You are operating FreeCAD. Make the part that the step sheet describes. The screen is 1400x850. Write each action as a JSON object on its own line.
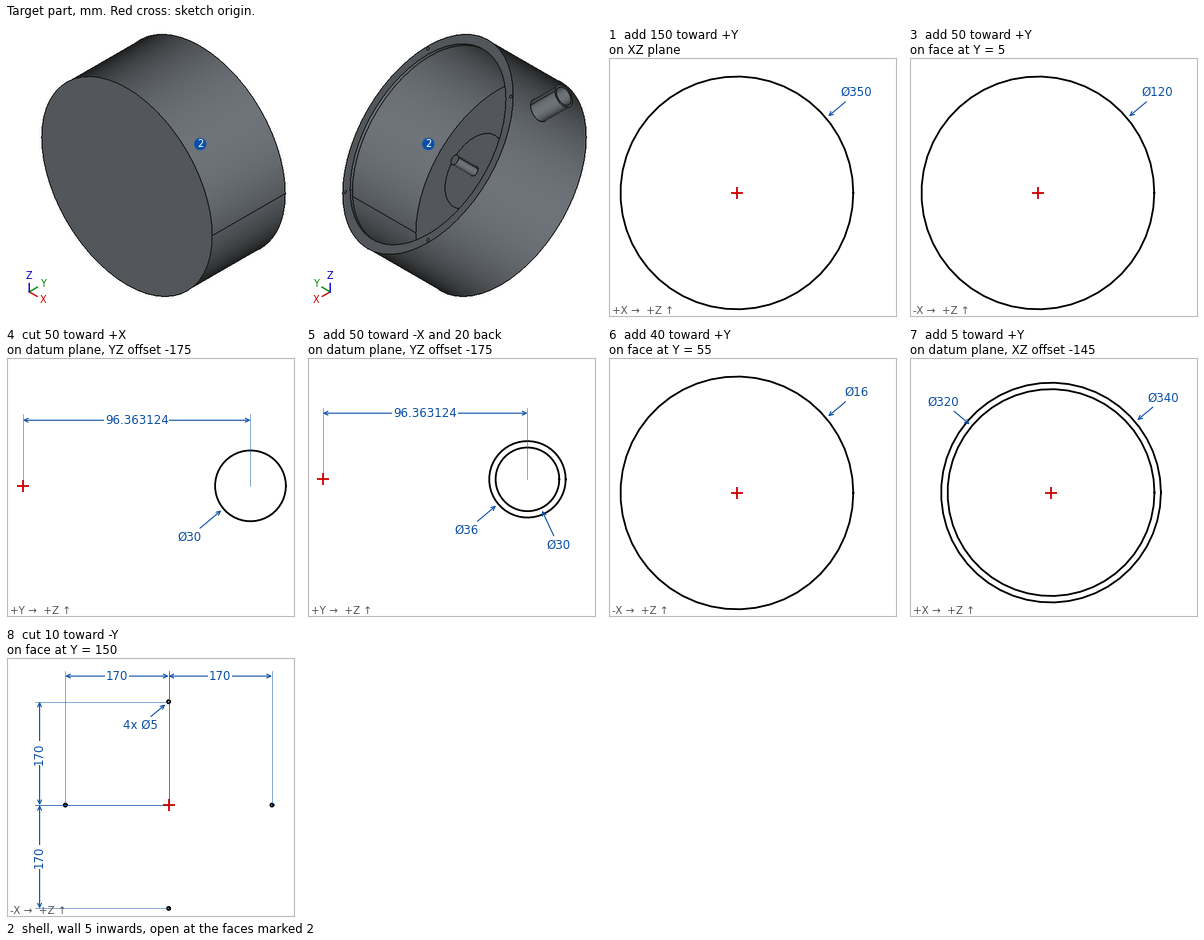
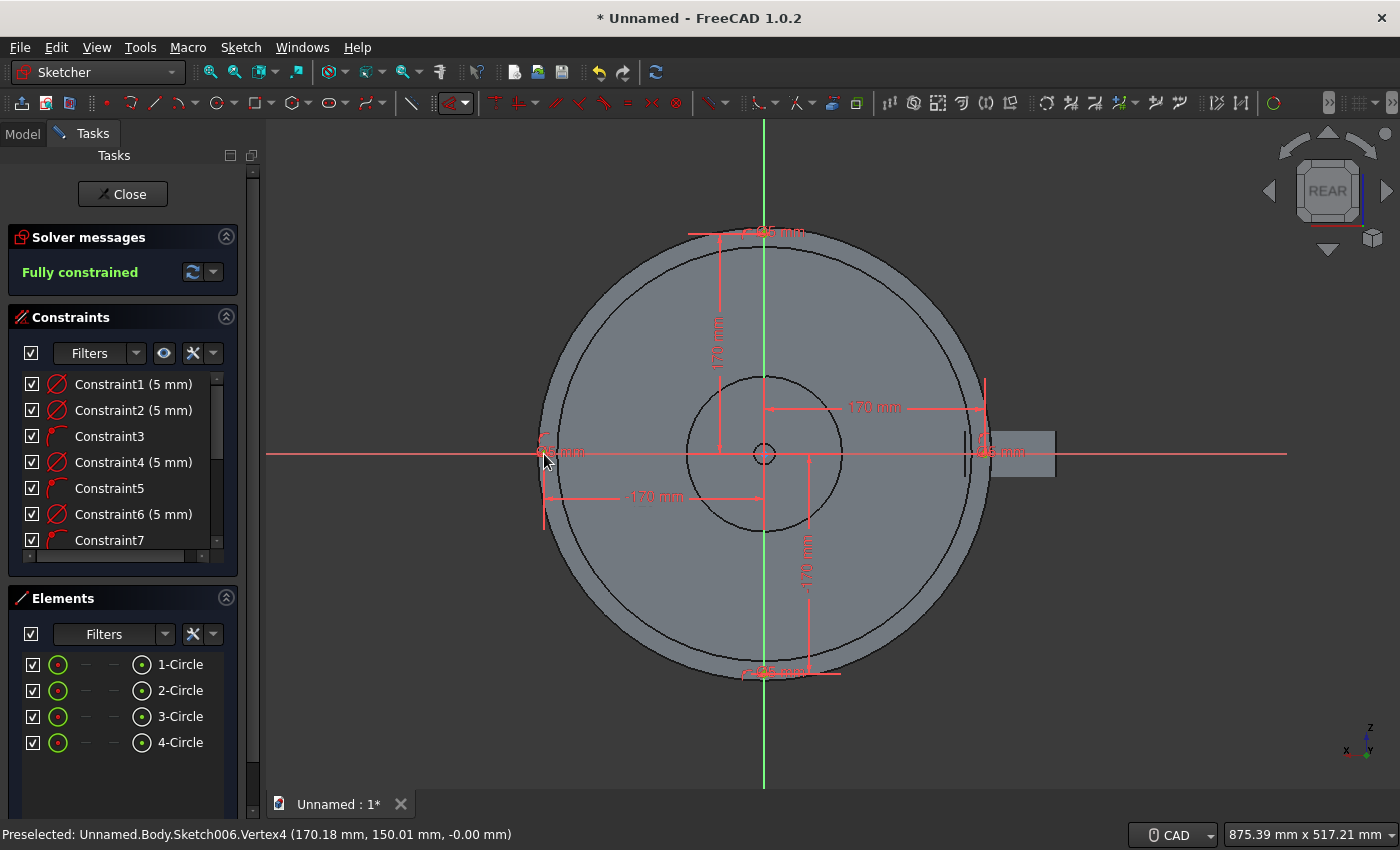
{"action": "left_click", "coordinate": [123, 194]}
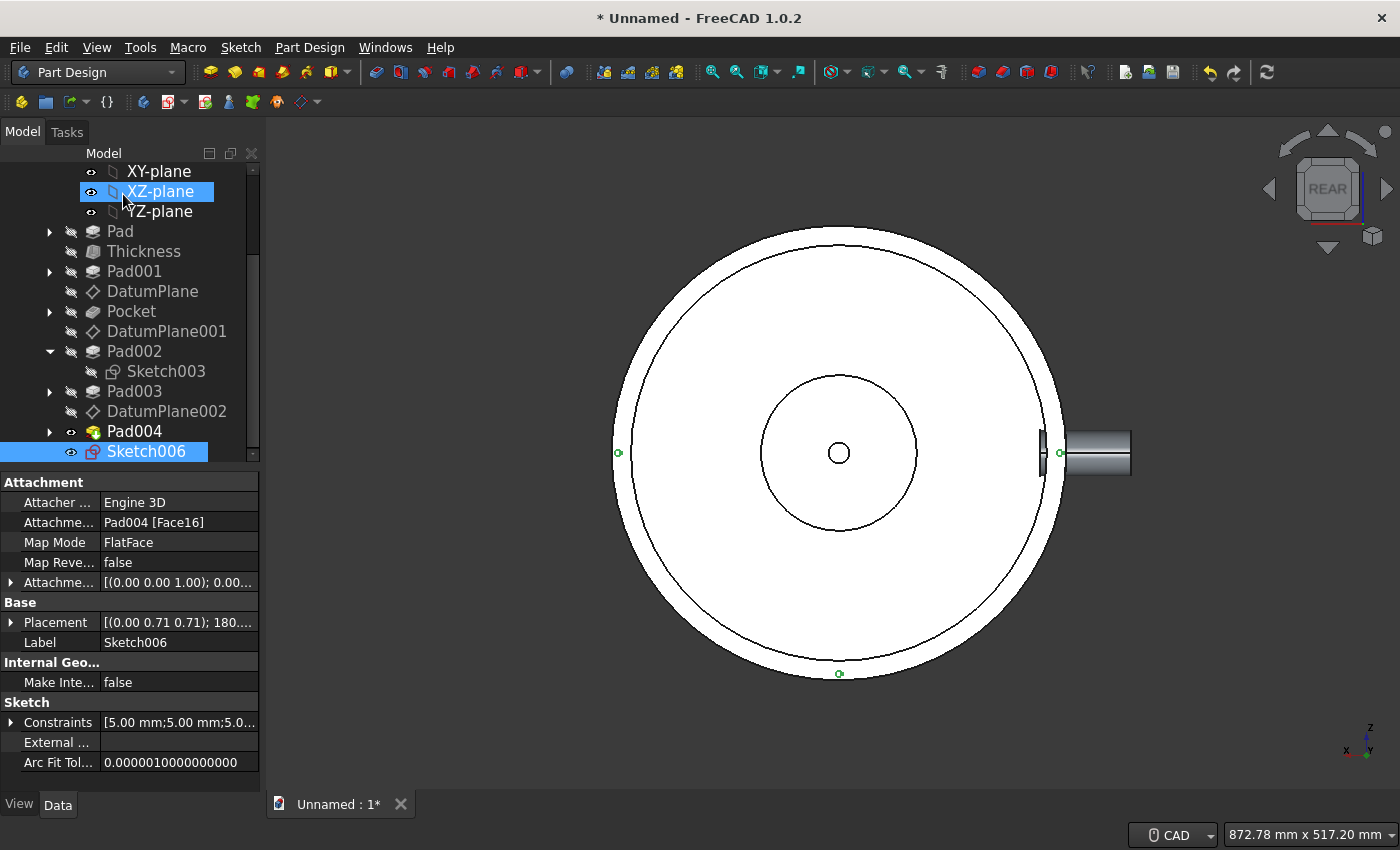
{"action": "left_click", "coordinate": [378, 72]}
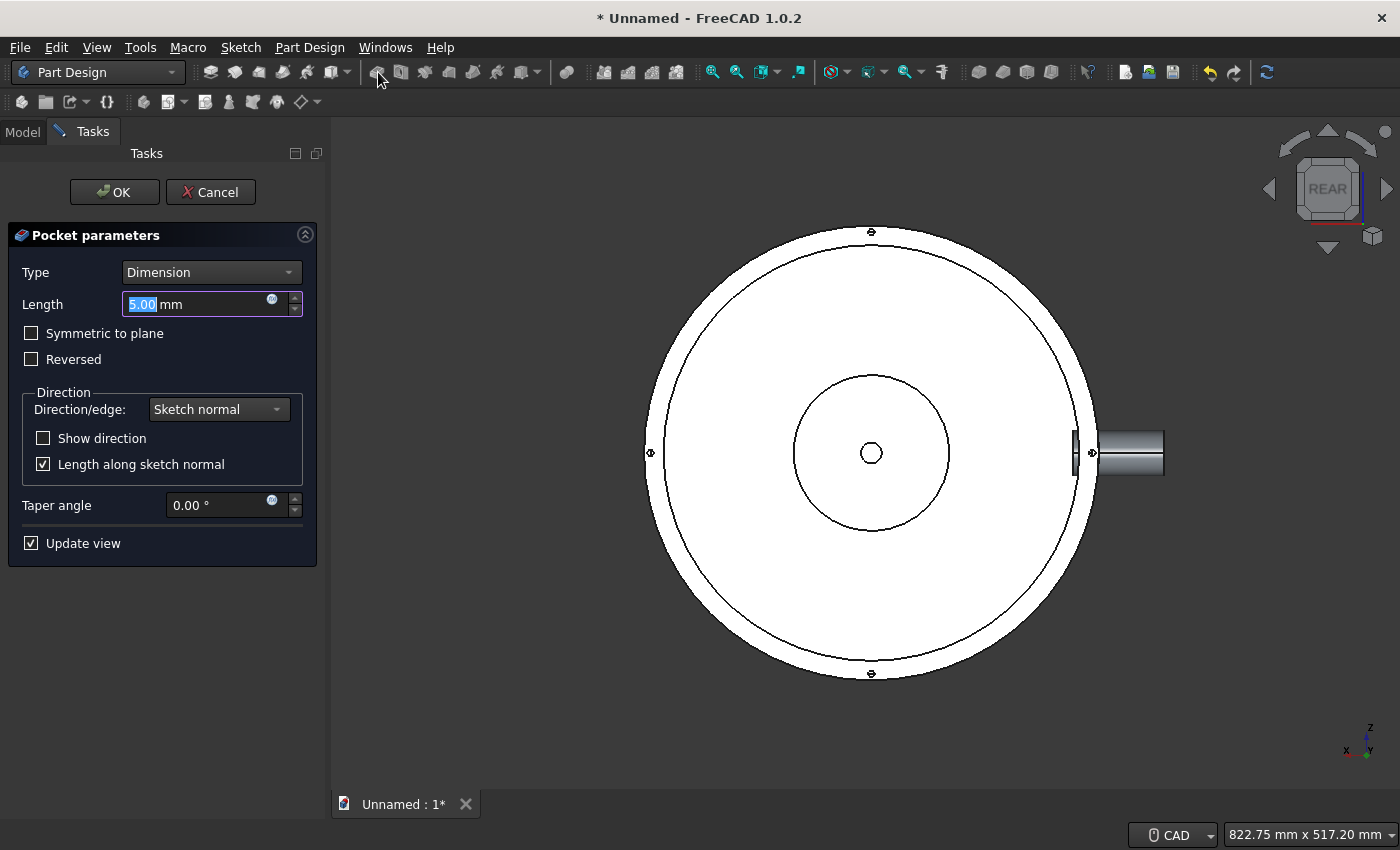
{"action": "type", "text": "10"}
{"action": "key", "text": "Tab"}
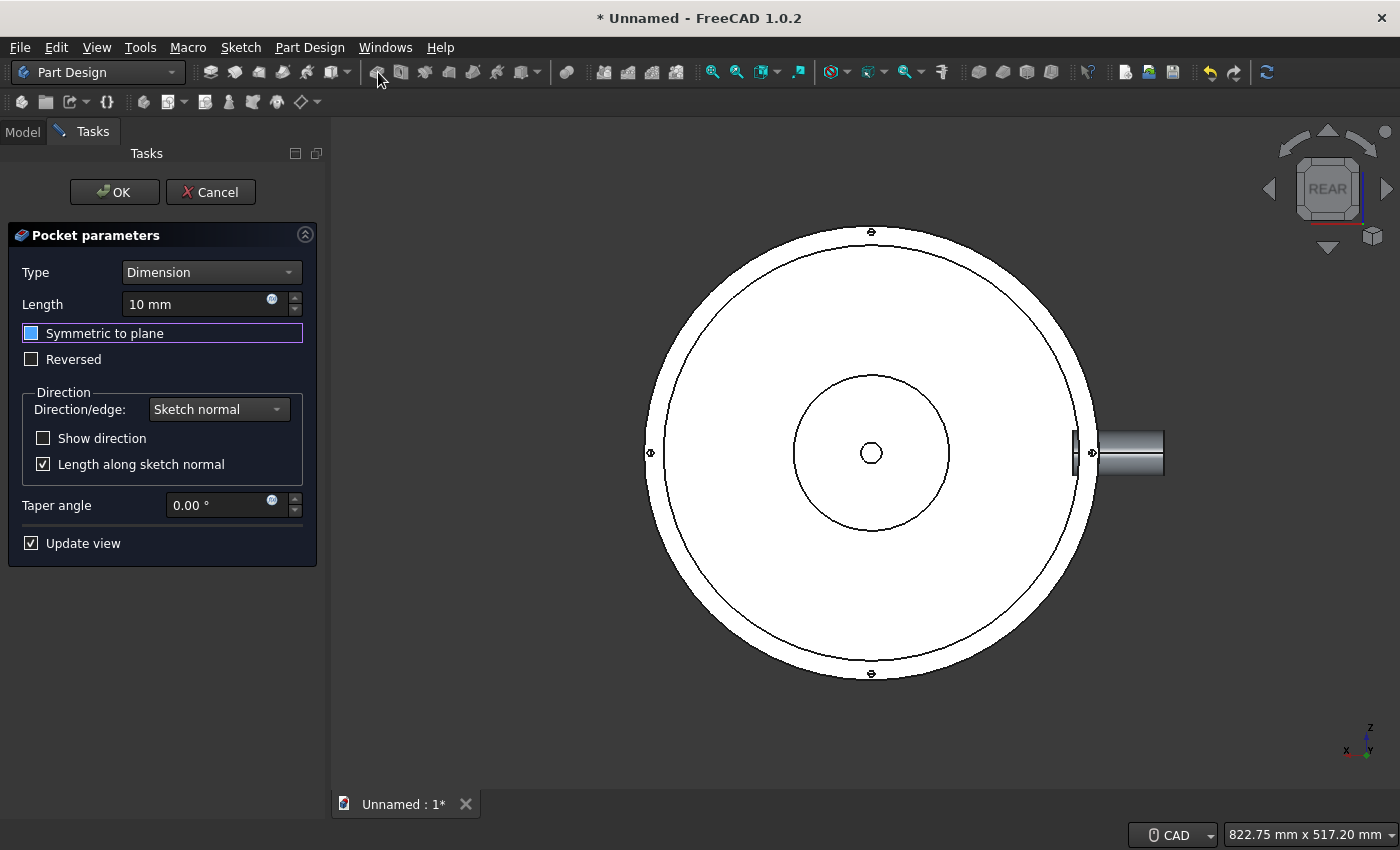
{"action": "left_click", "coordinate": [115, 192]}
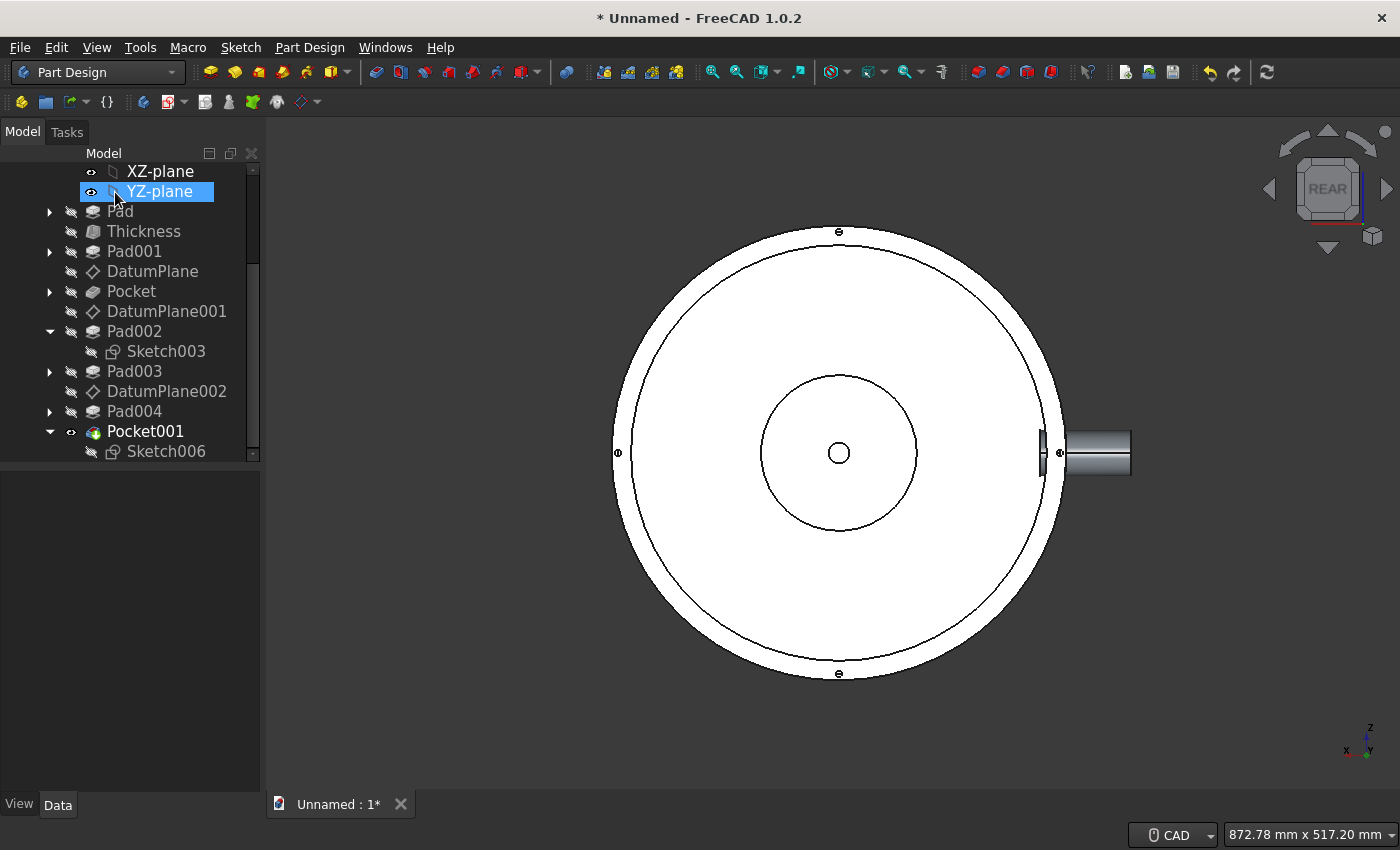
{"action": "key", "text": "0"}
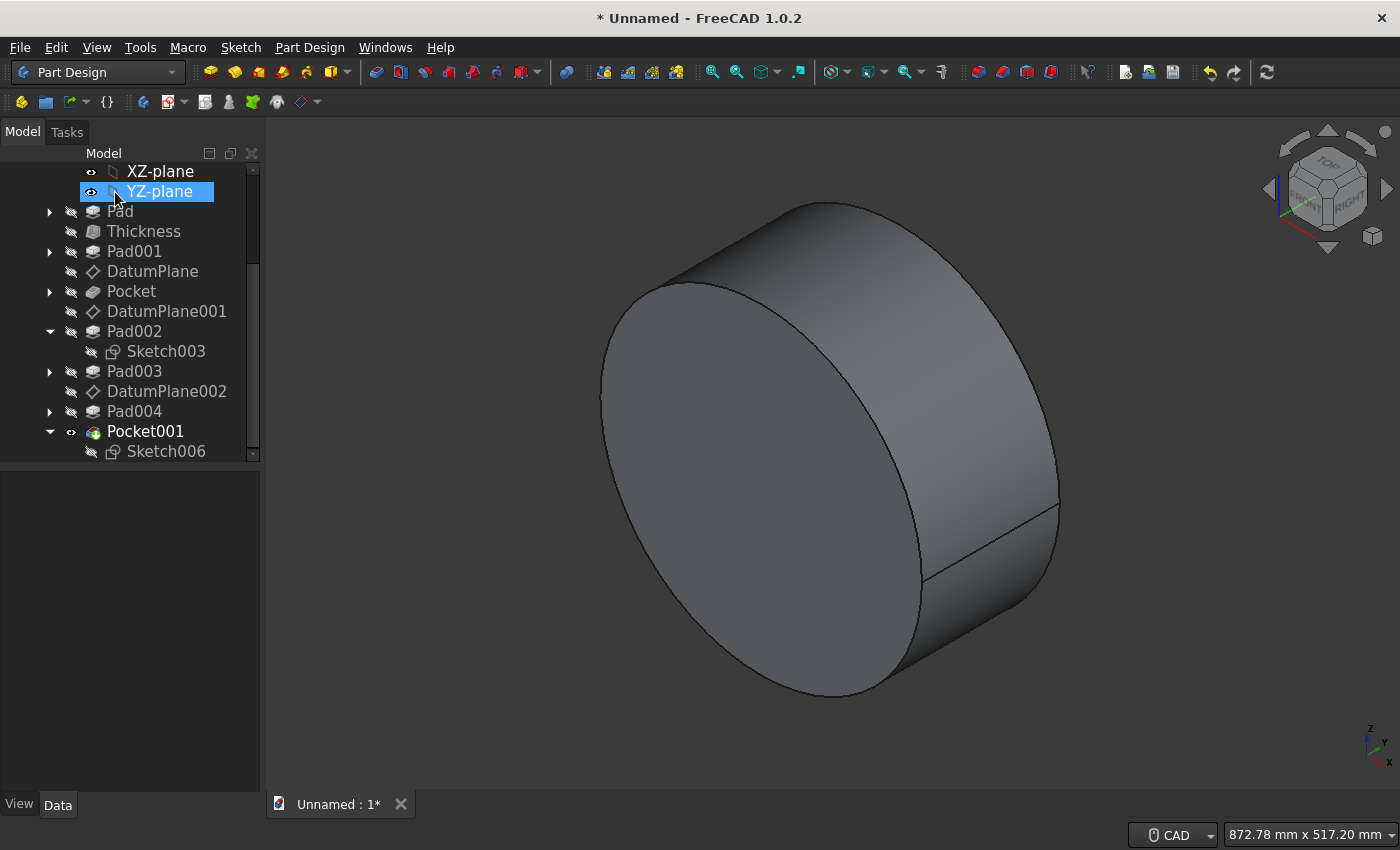
{"action": "left_click", "coordinate": [714, 72]}